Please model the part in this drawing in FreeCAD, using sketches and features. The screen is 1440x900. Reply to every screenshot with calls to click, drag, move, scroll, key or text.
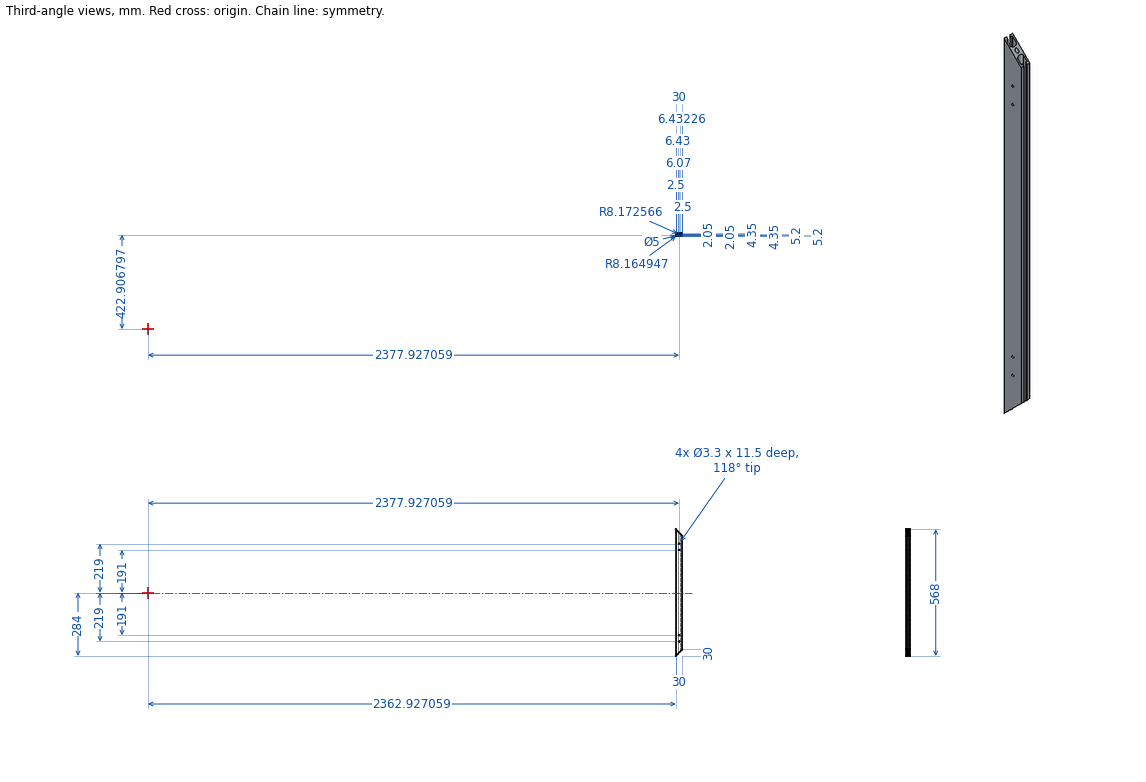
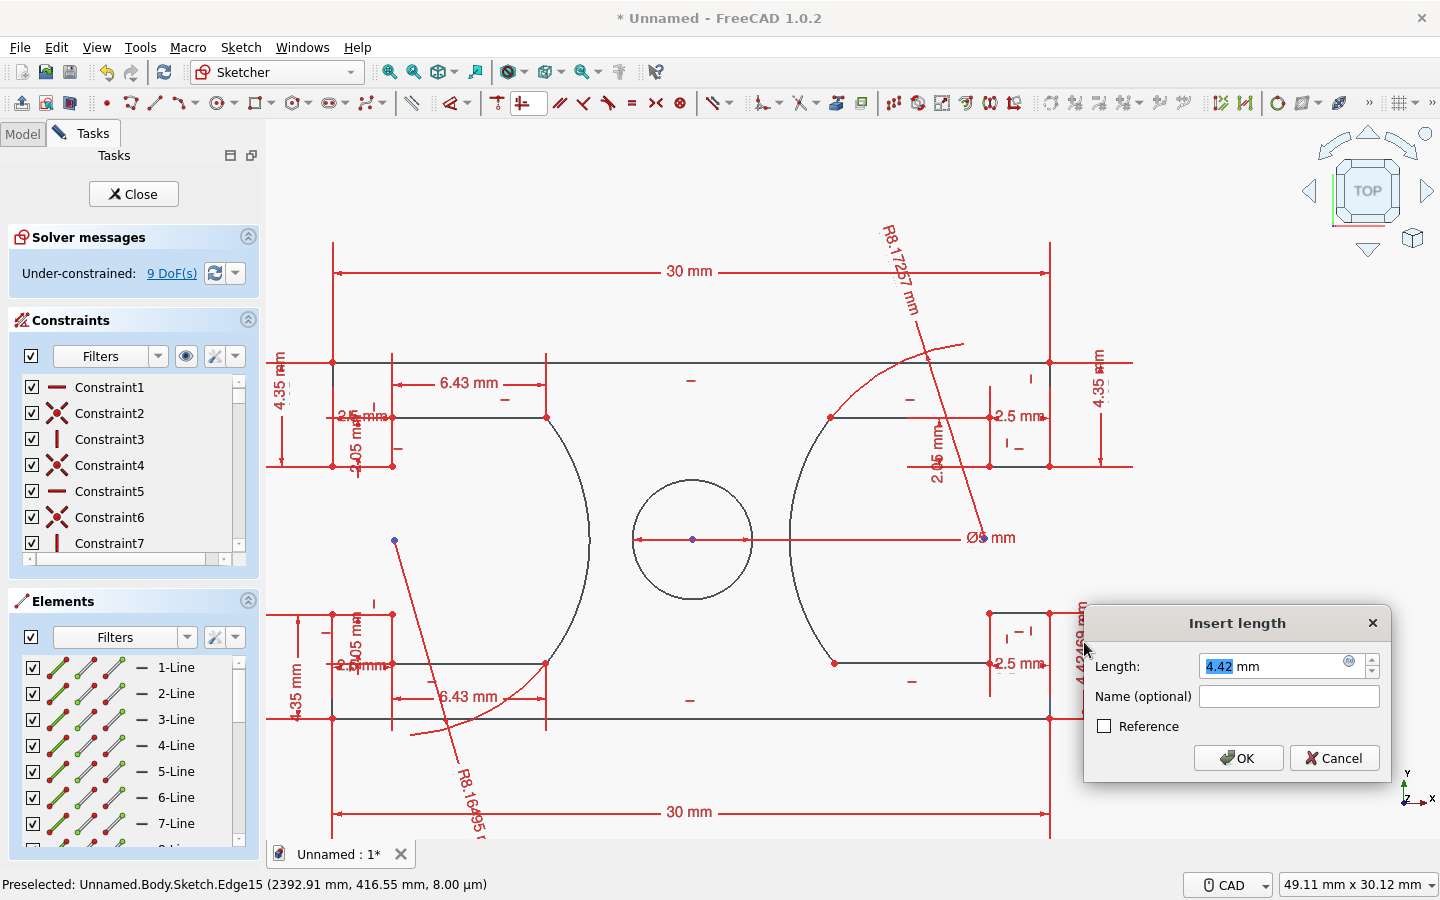
text(4.35)
key(Return)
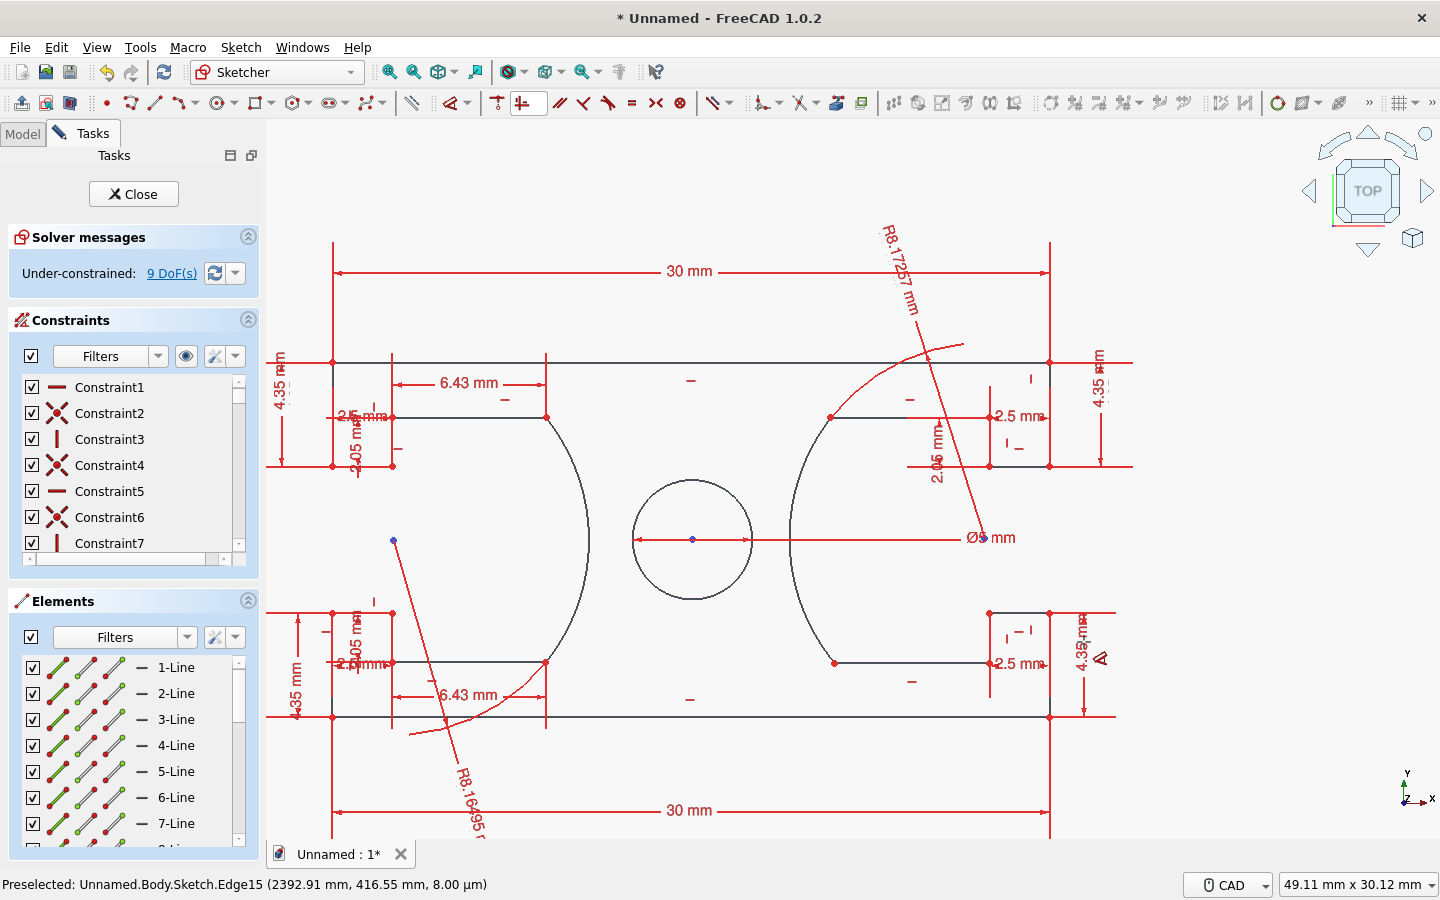
click(990, 628)
click(956, 638)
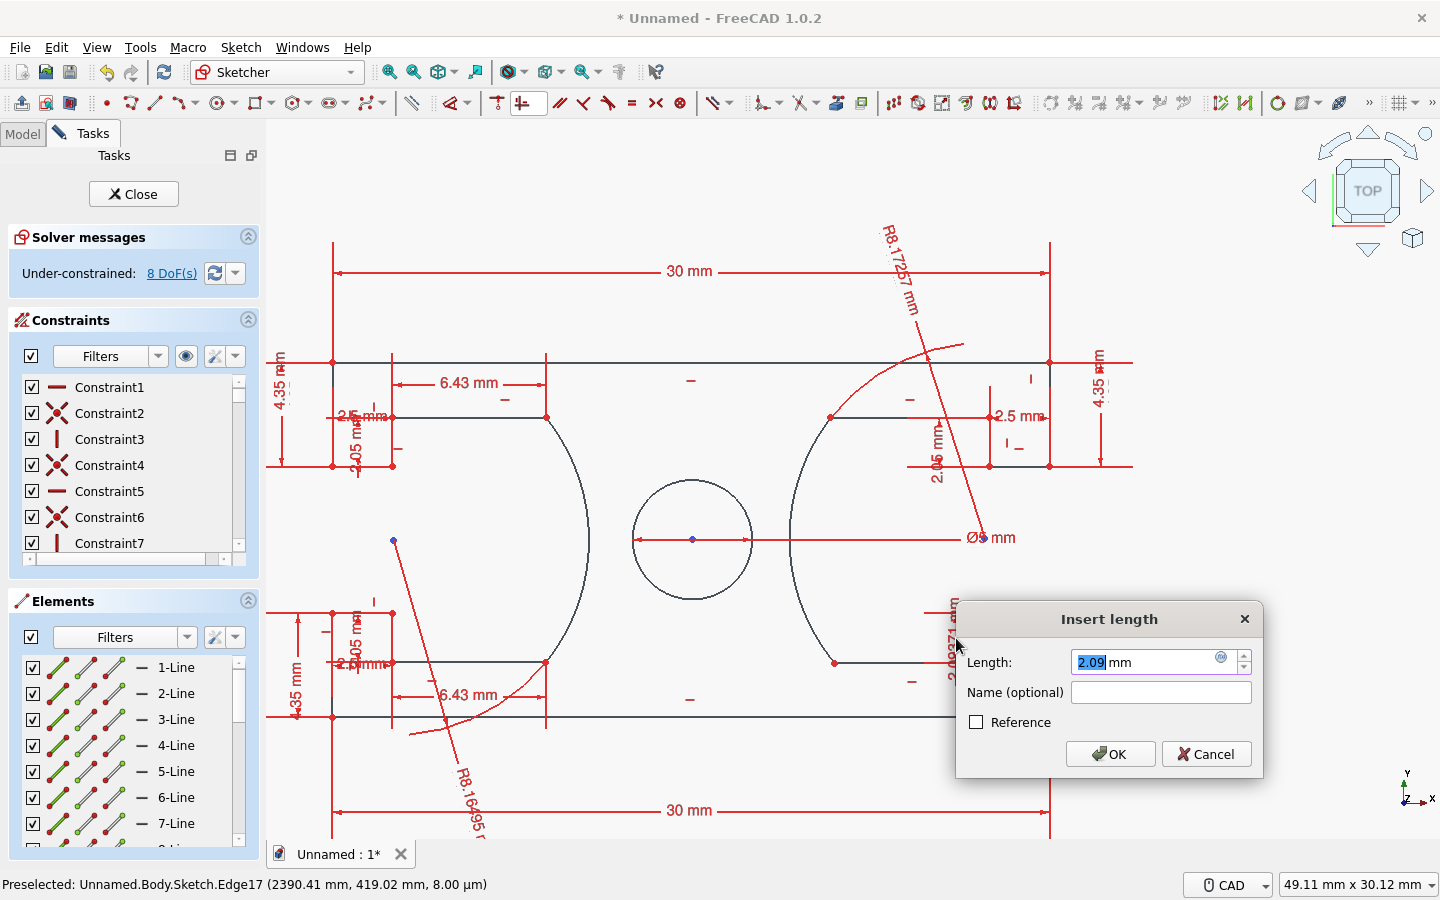
text(2.05)
key(Return)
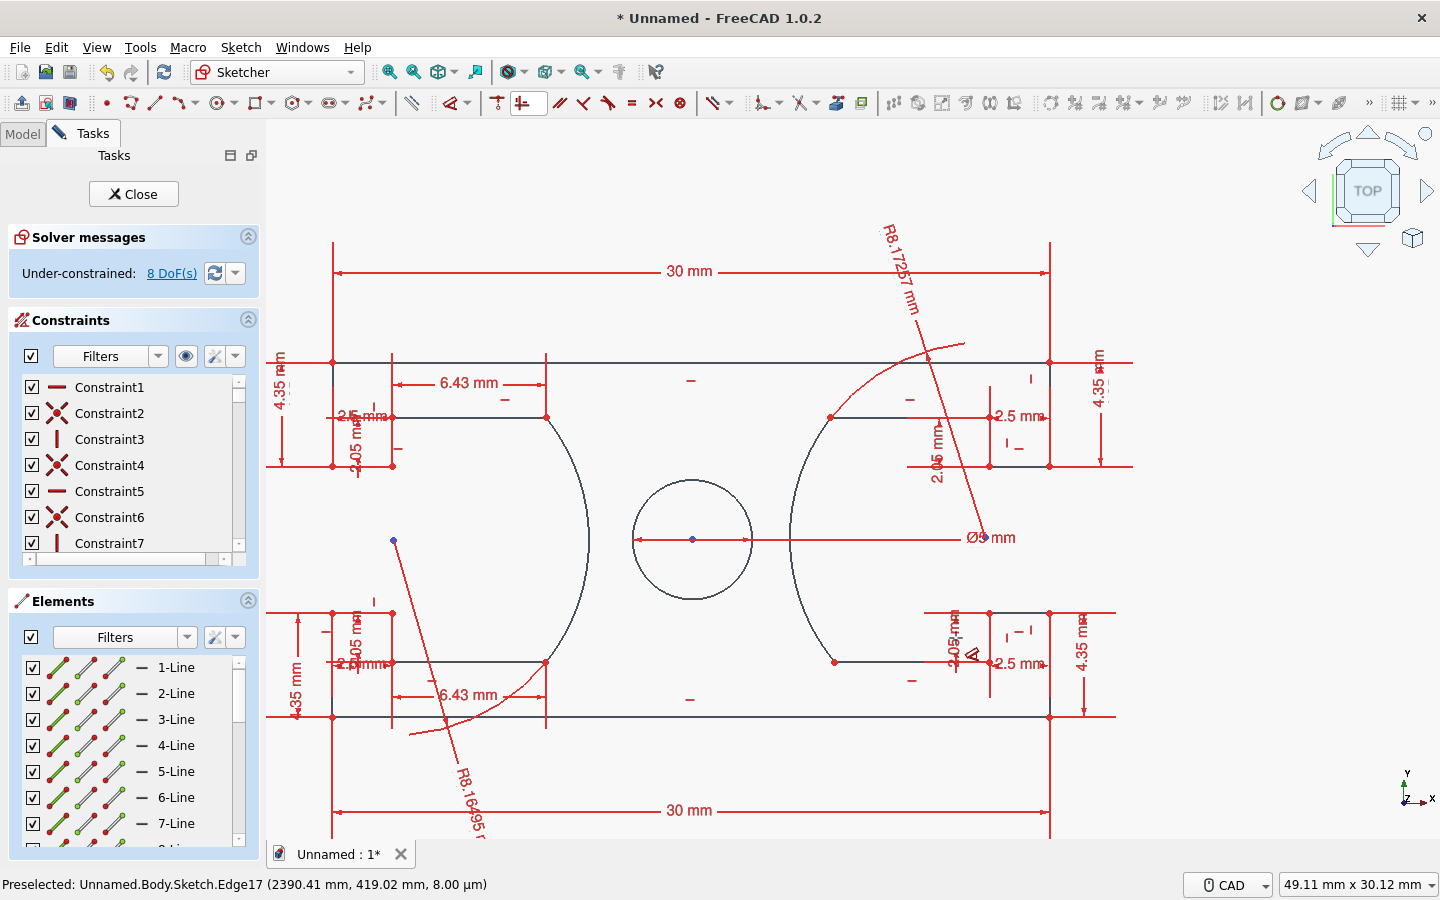
click(831, 418)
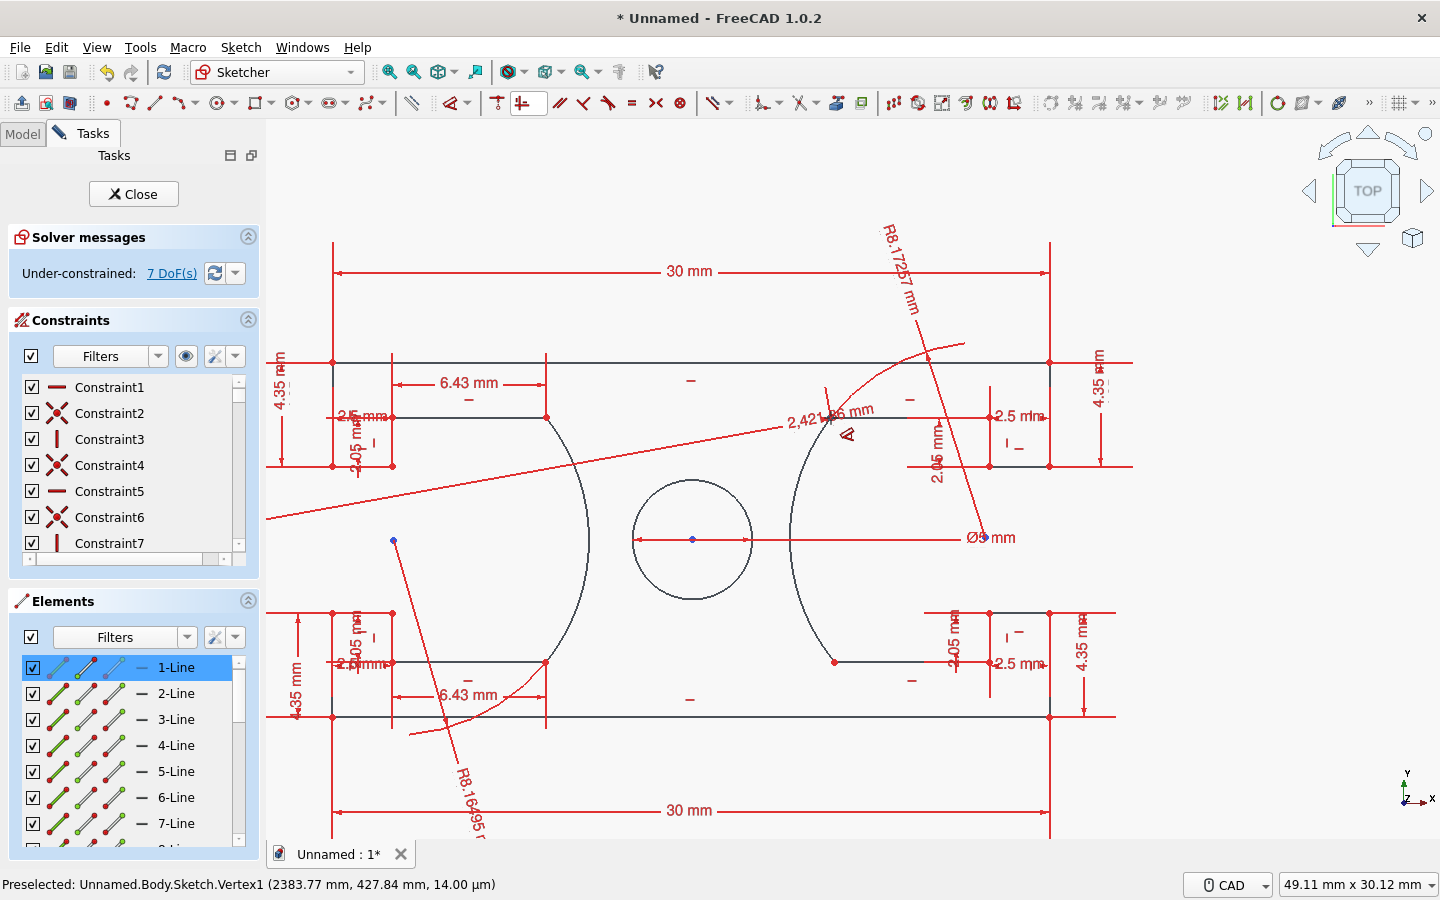
click(692, 540)
click(865, 479)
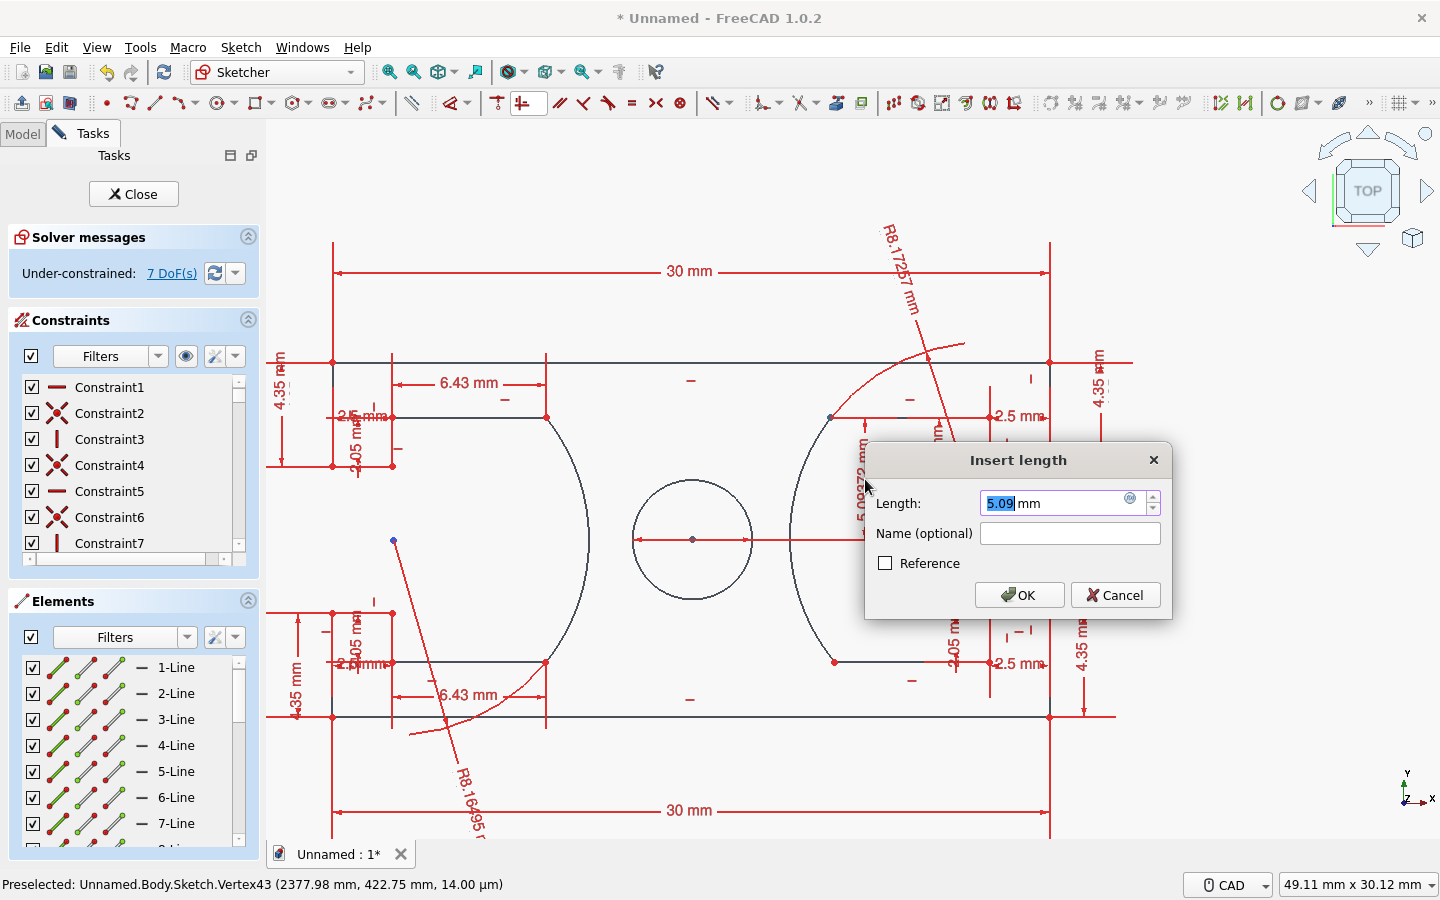
text(5.2)
key(Return)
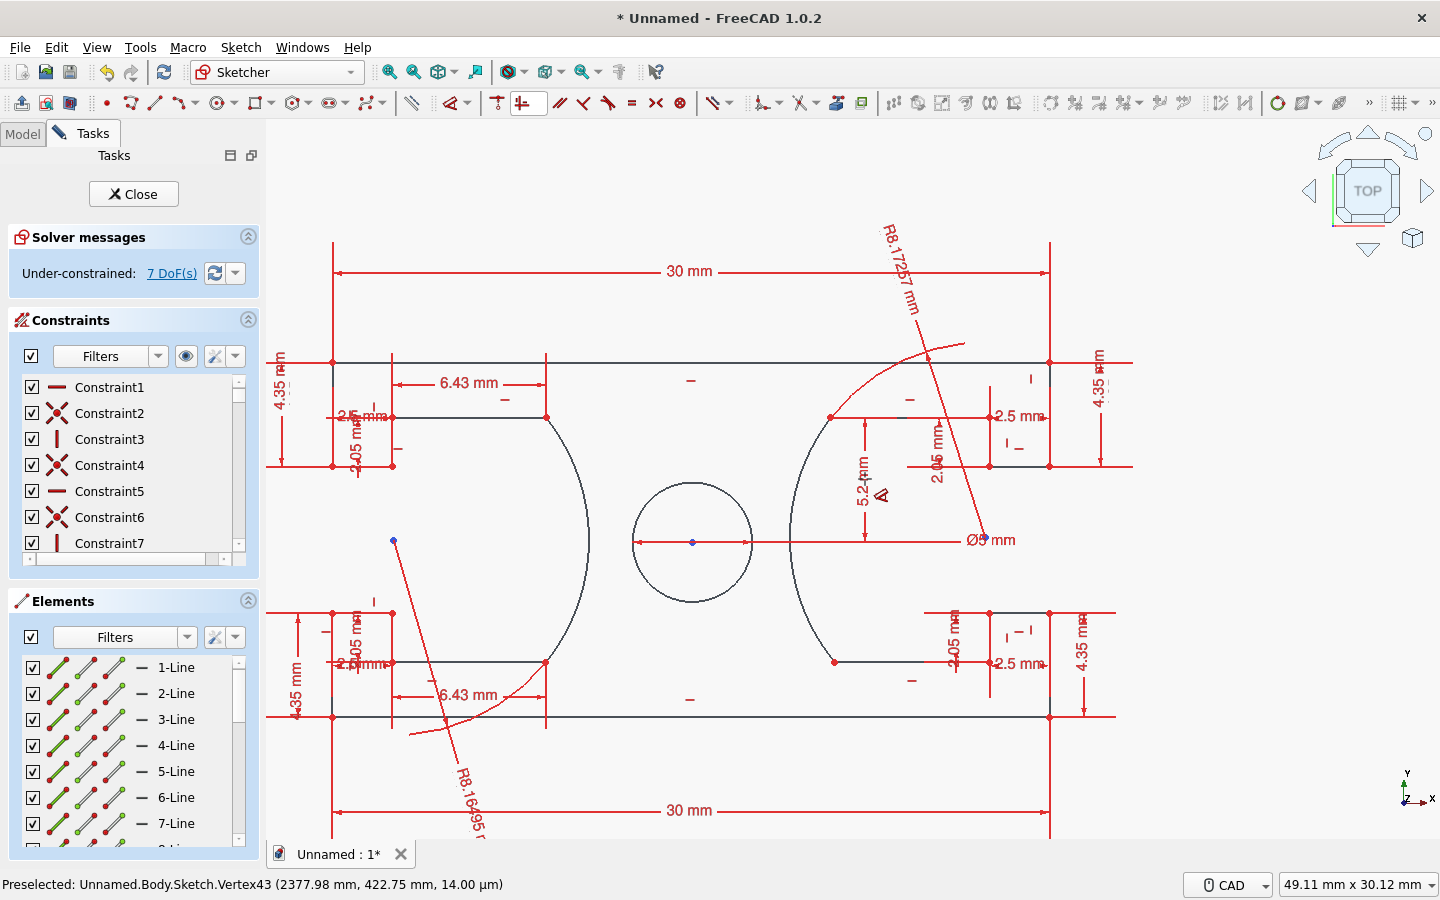
click(835, 662)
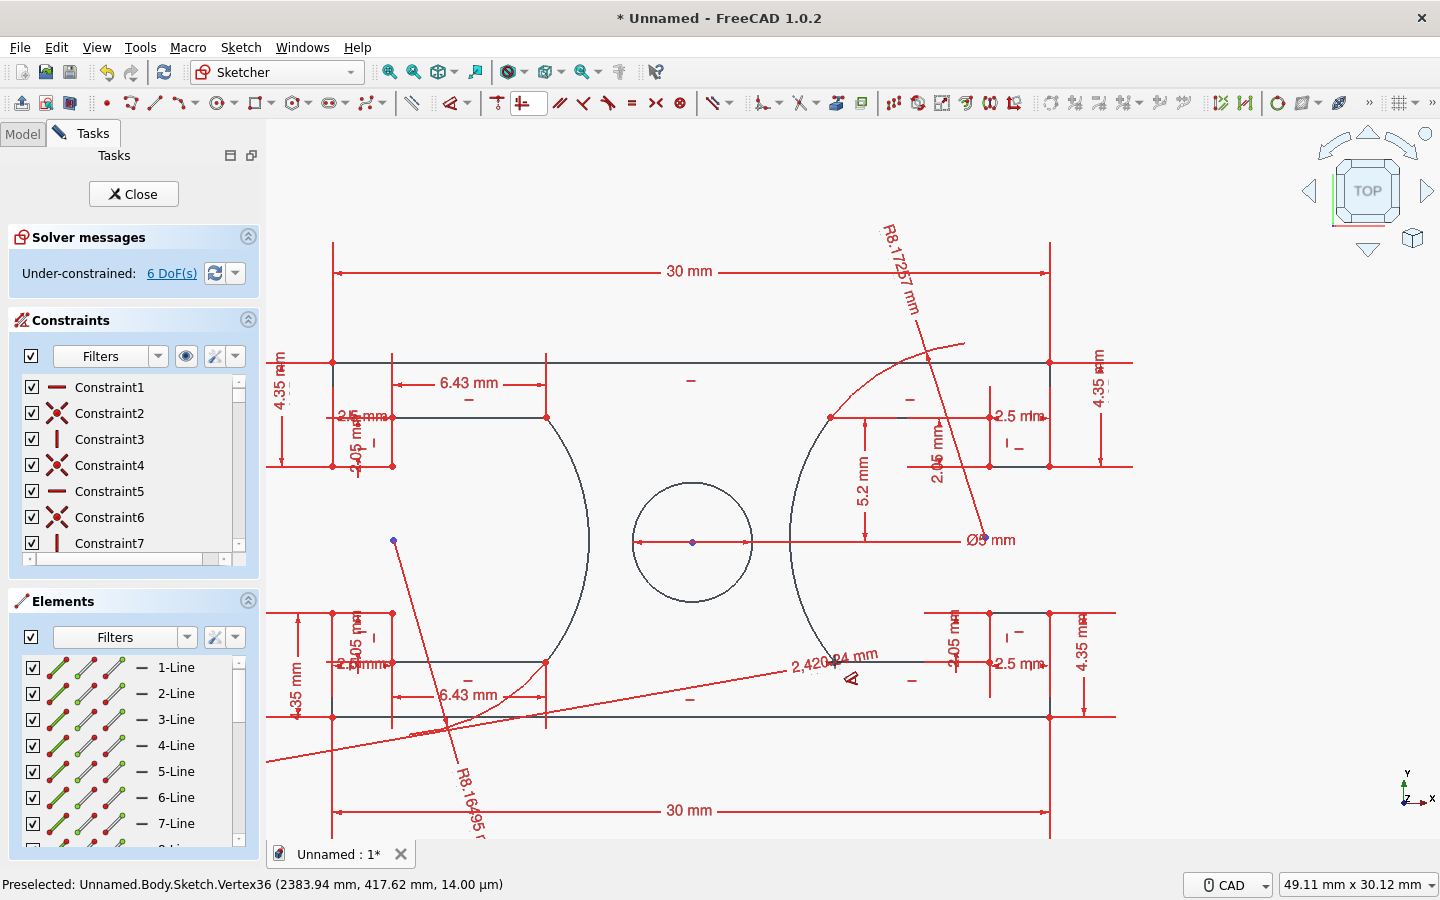
click(692, 542)
click(869, 602)